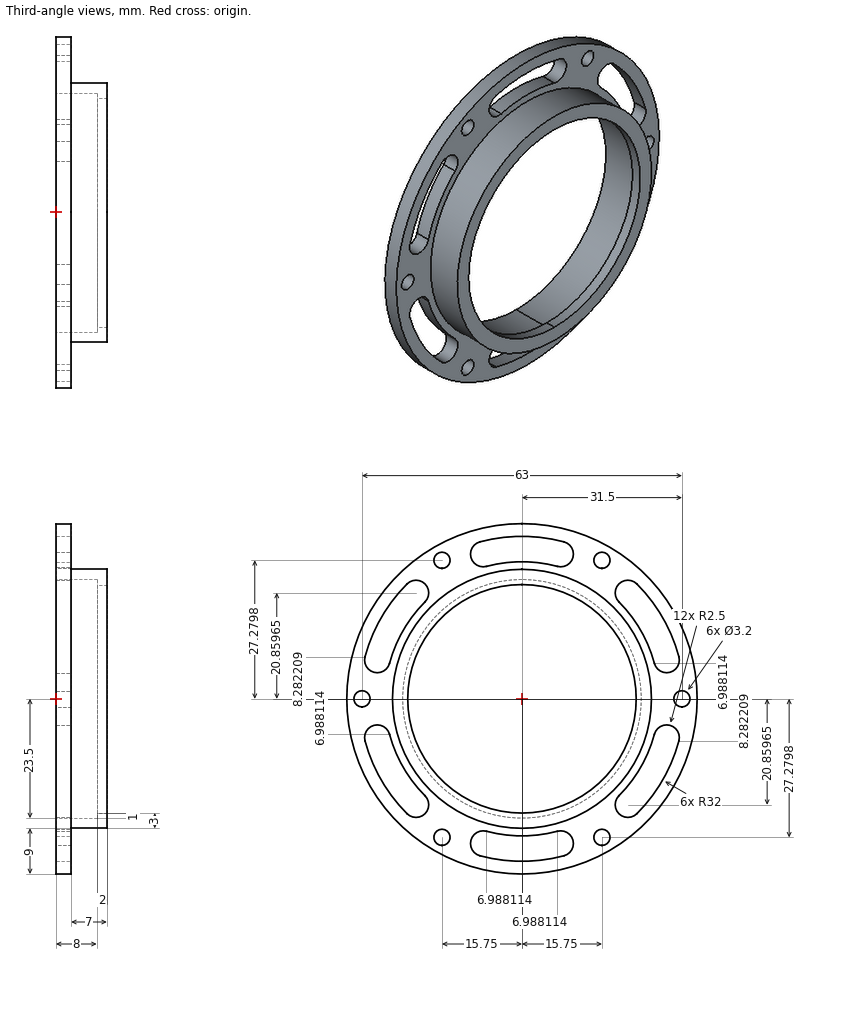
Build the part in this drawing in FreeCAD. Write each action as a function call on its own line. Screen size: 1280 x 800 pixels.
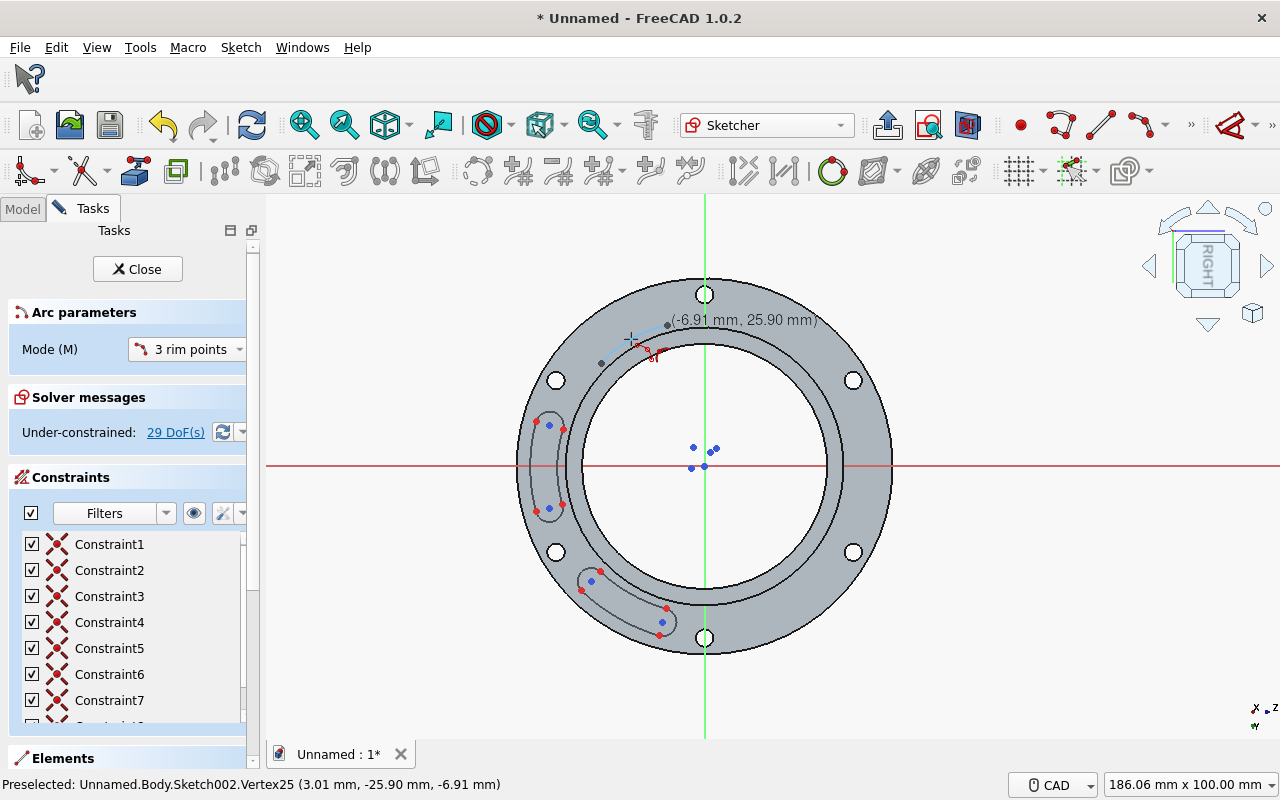
click(660, 298)
click(676, 308)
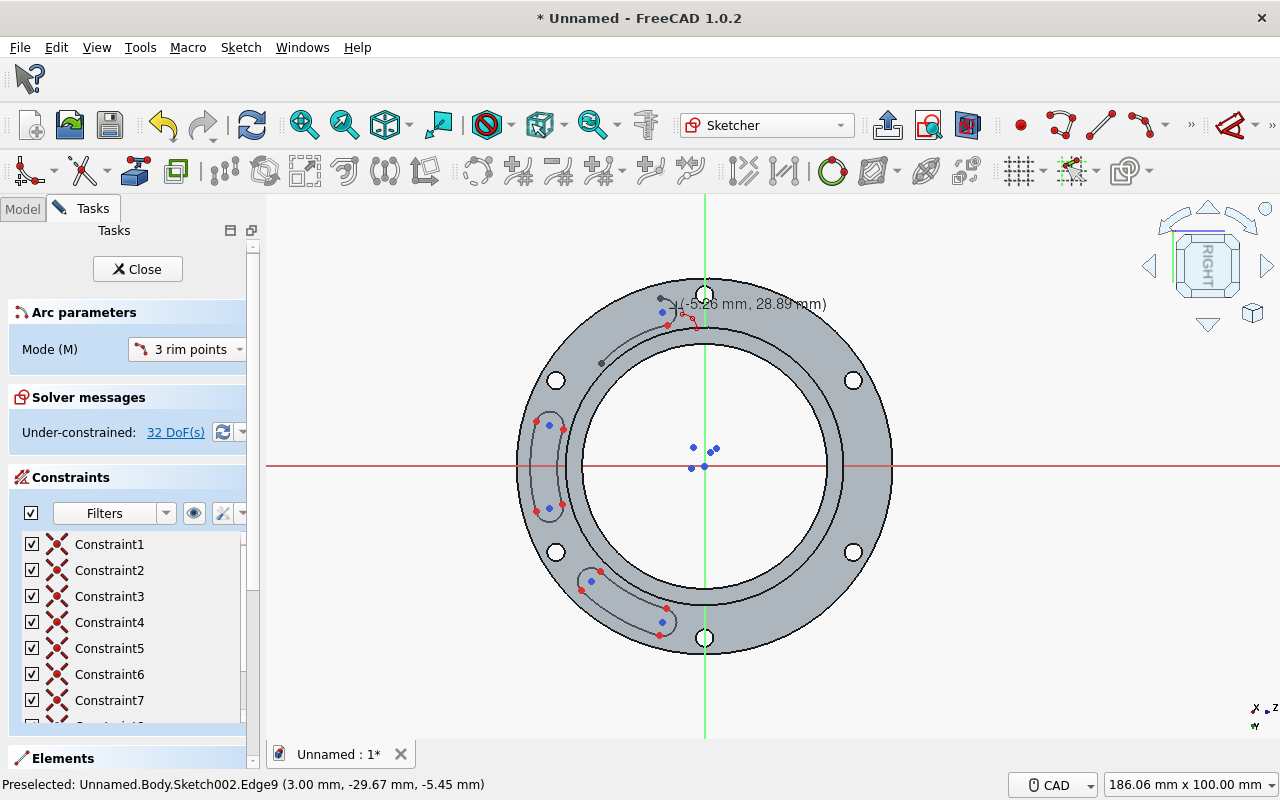
click(660, 299)
click(581, 343)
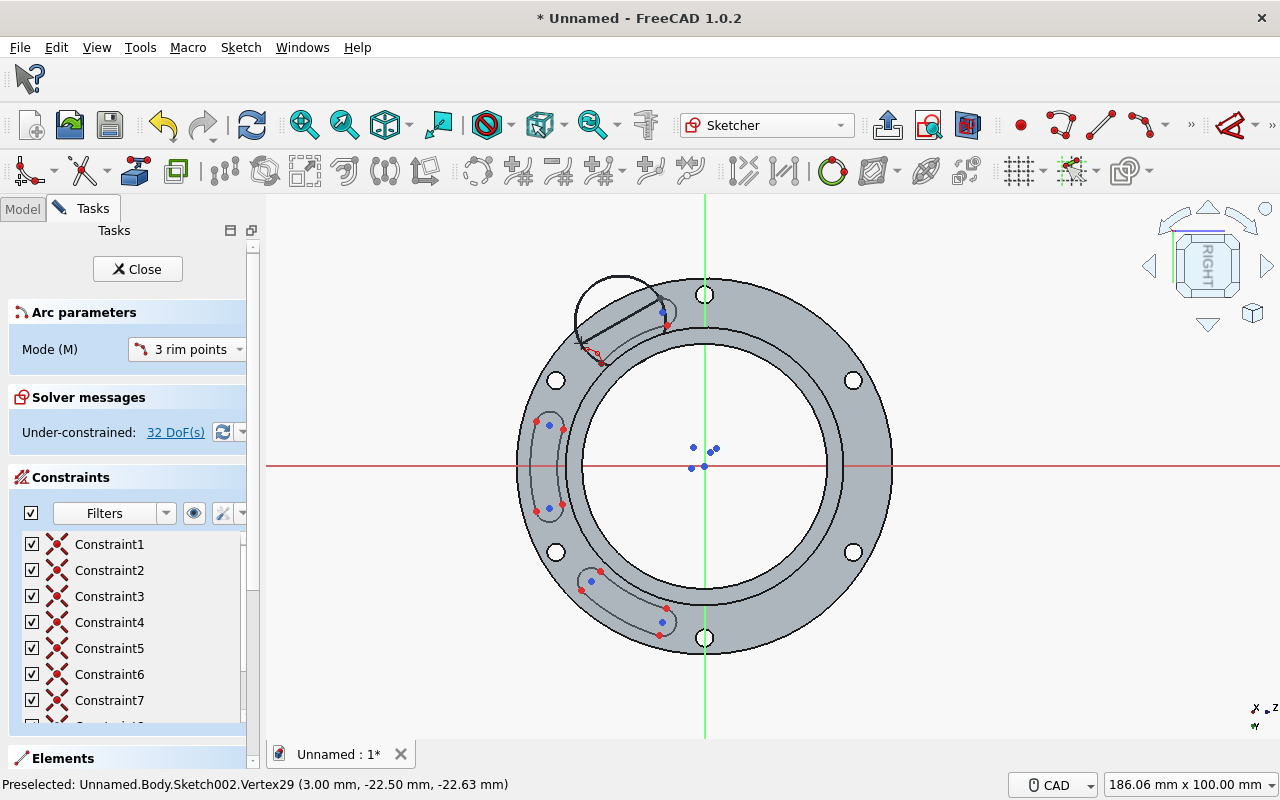
scroll(617, 315, up, 5)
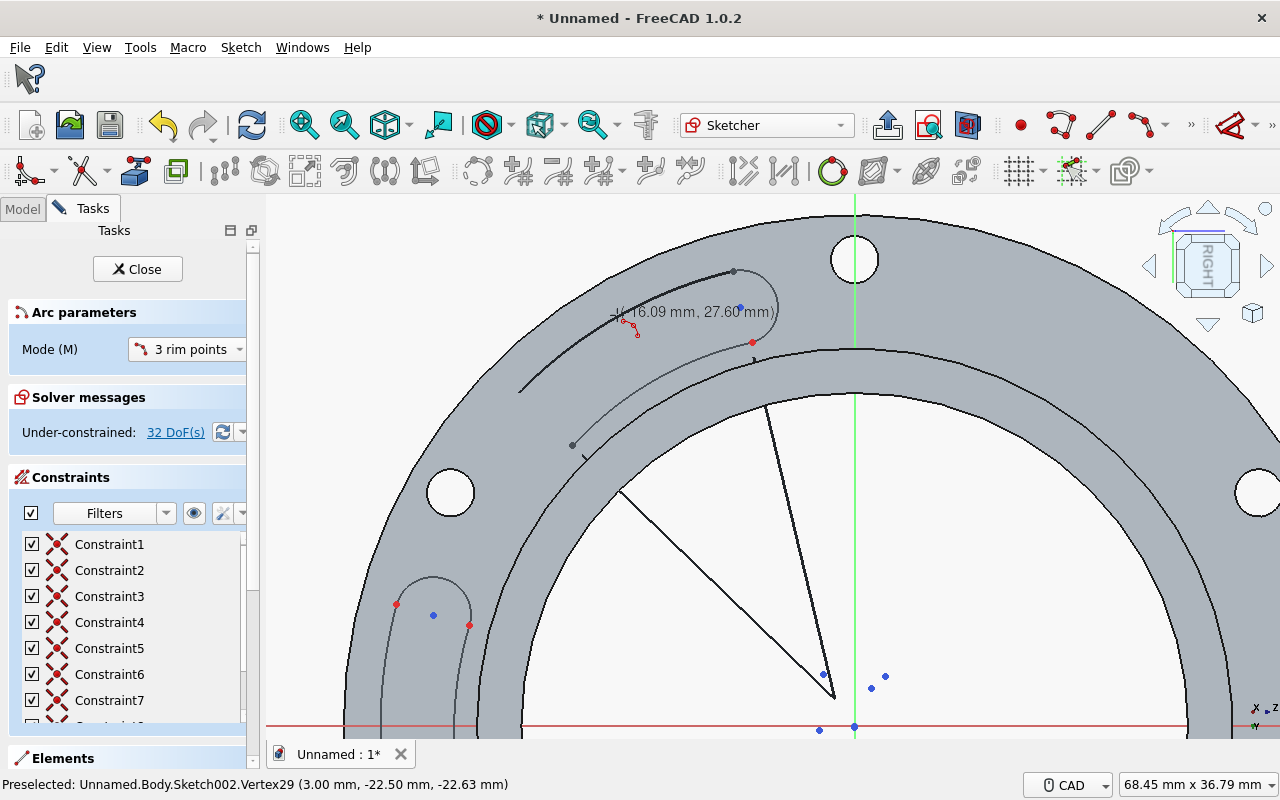
click(618, 316)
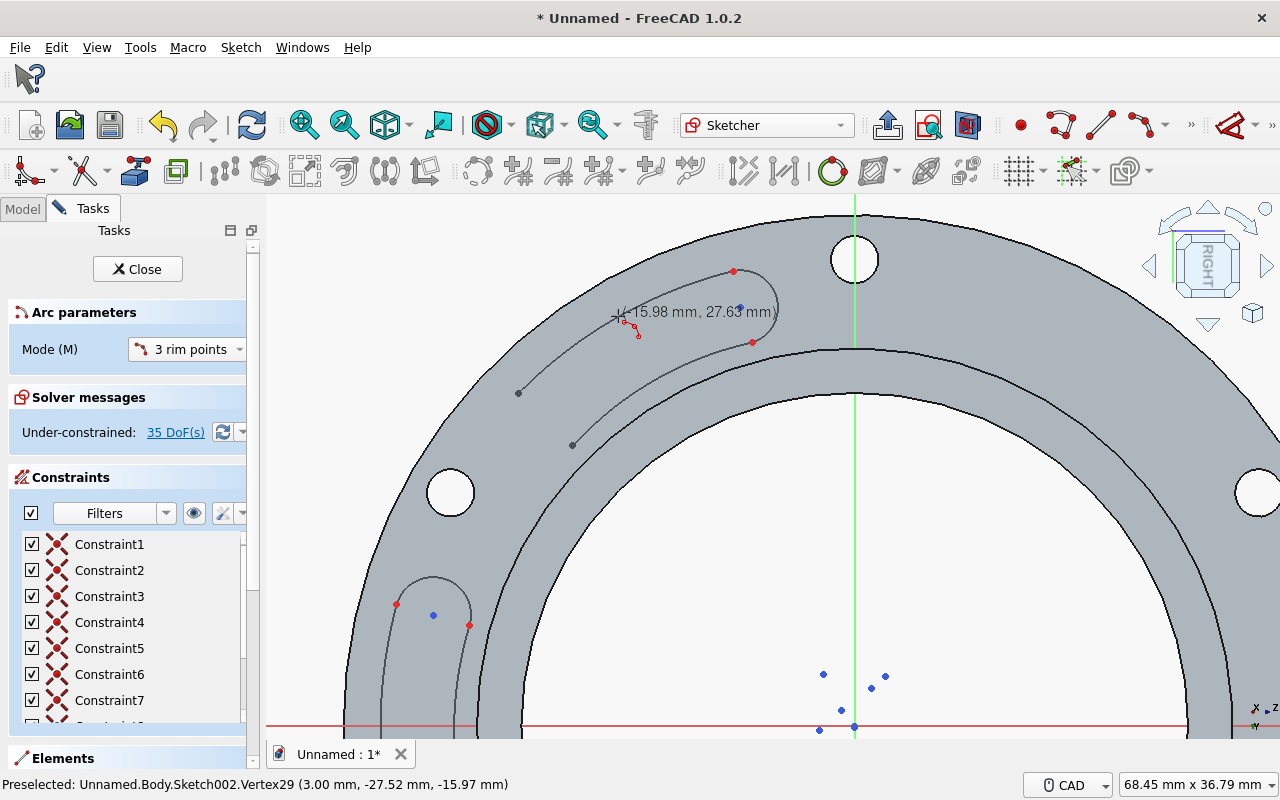
click(519, 393)
click(573, 446)
click(519, 443)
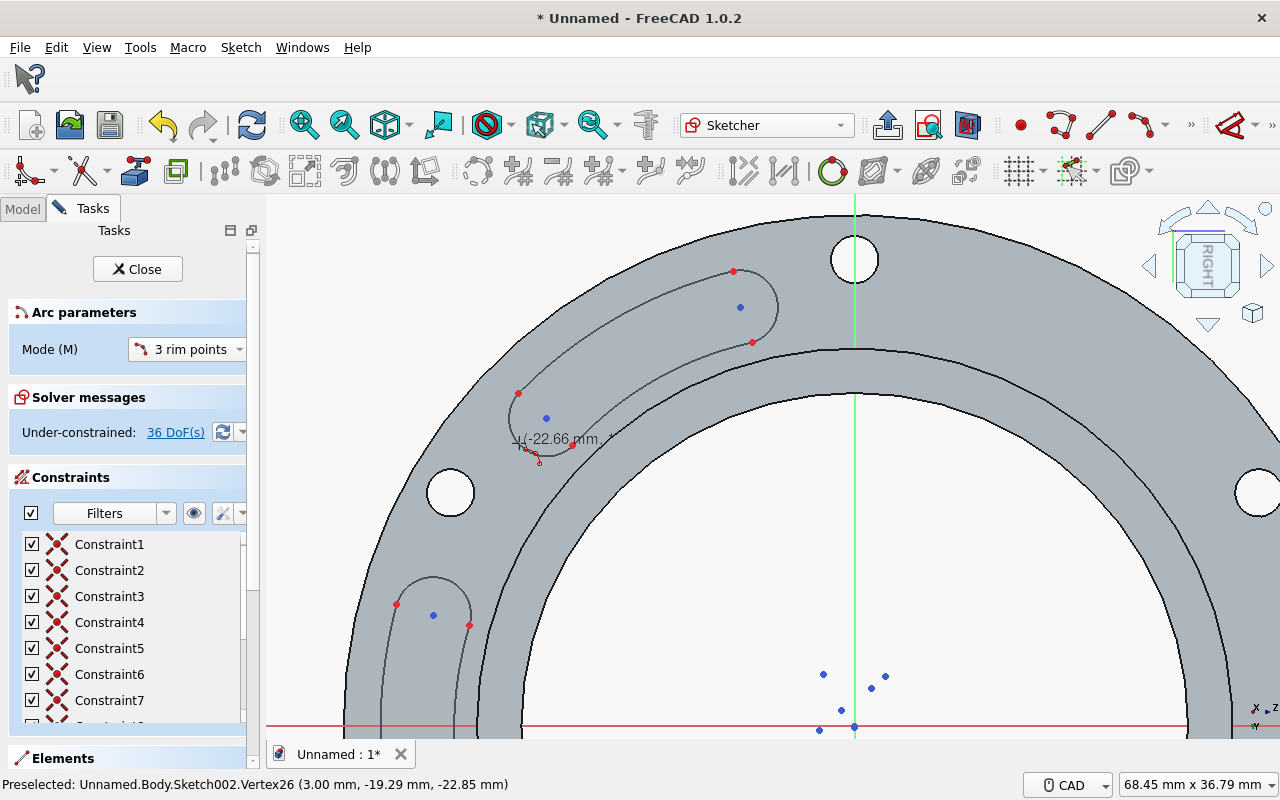
scroll(617, 315, down, 5)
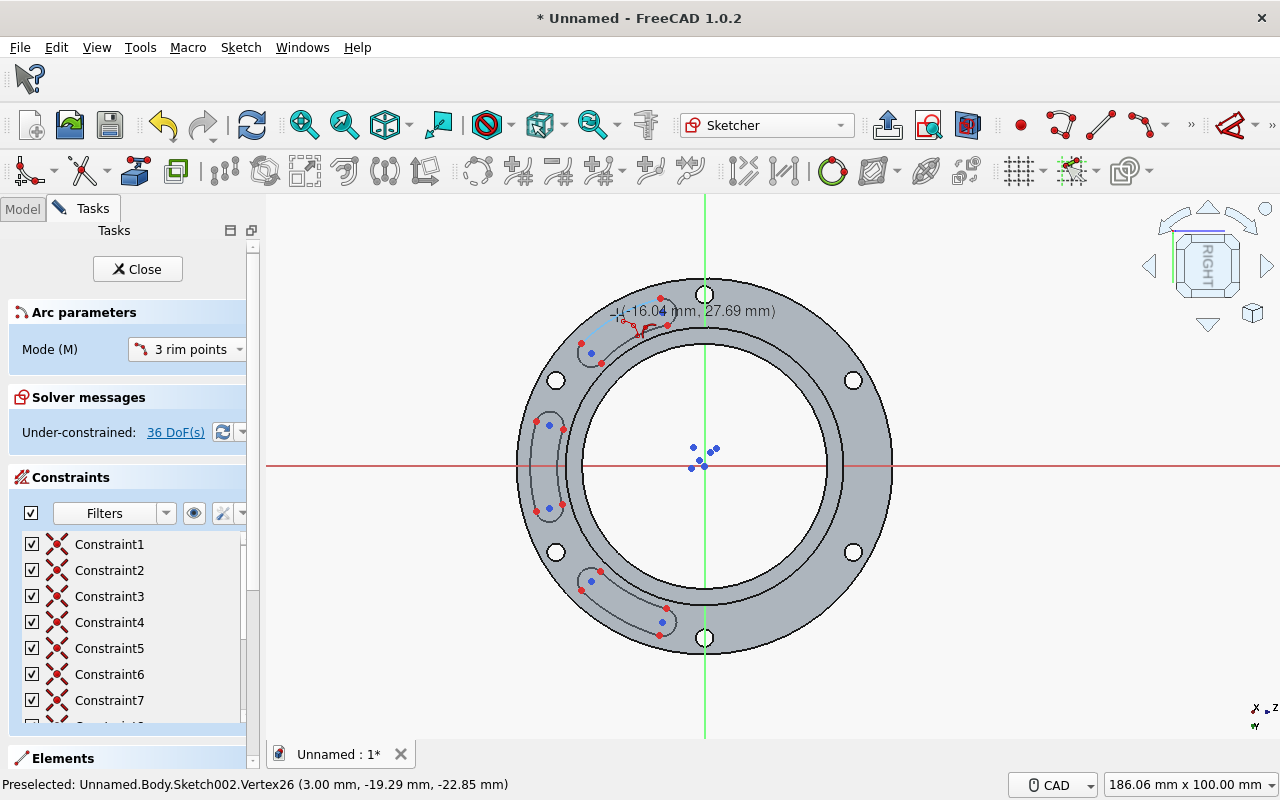
click(809, 362)
click(828, 343)
click(828, 362)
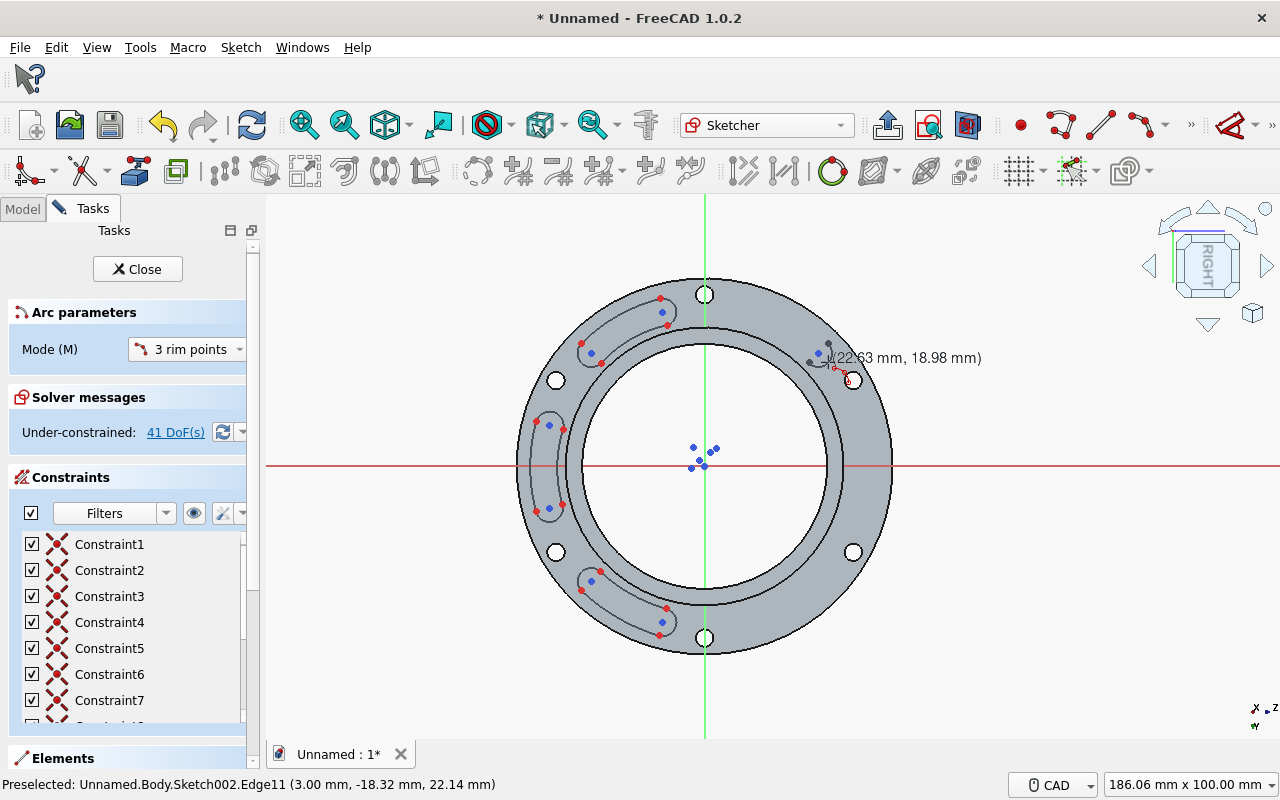
click(828, 344)
click(750, 298)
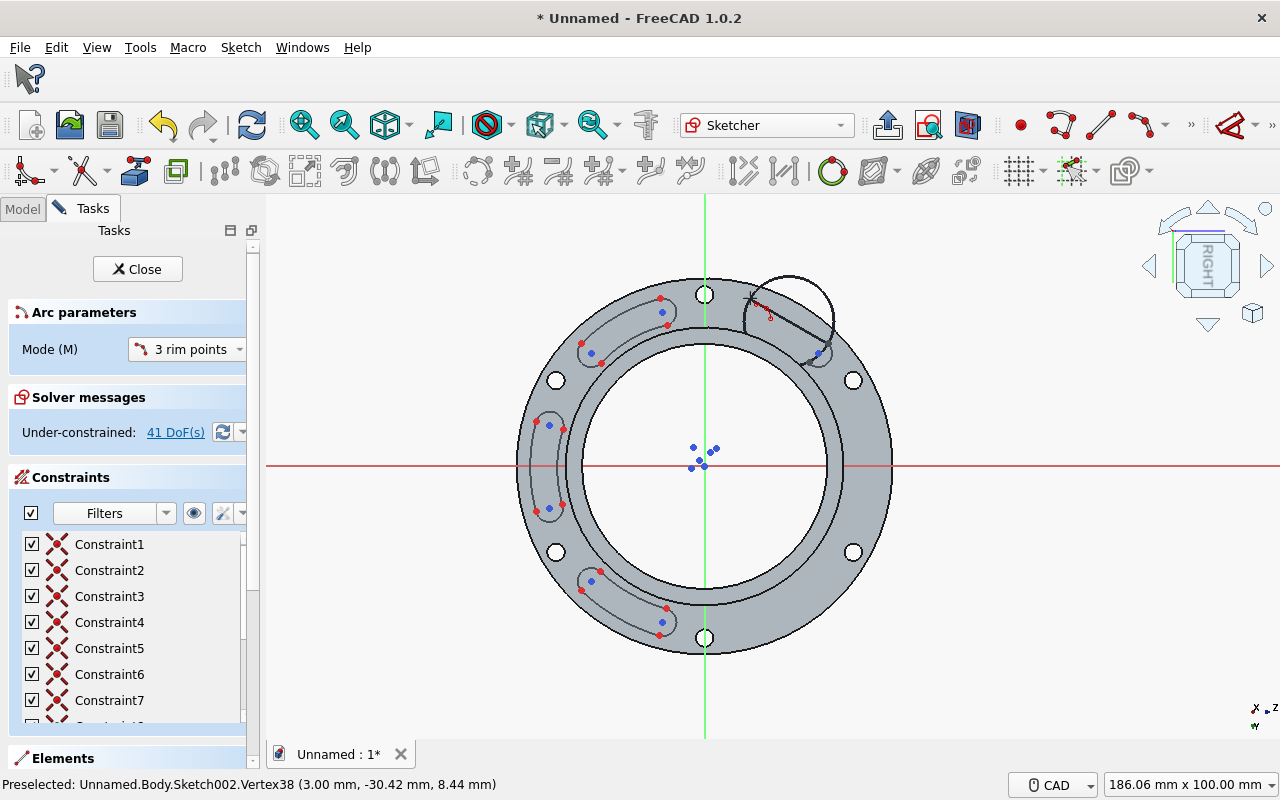
scroll(792, 315, up, 5)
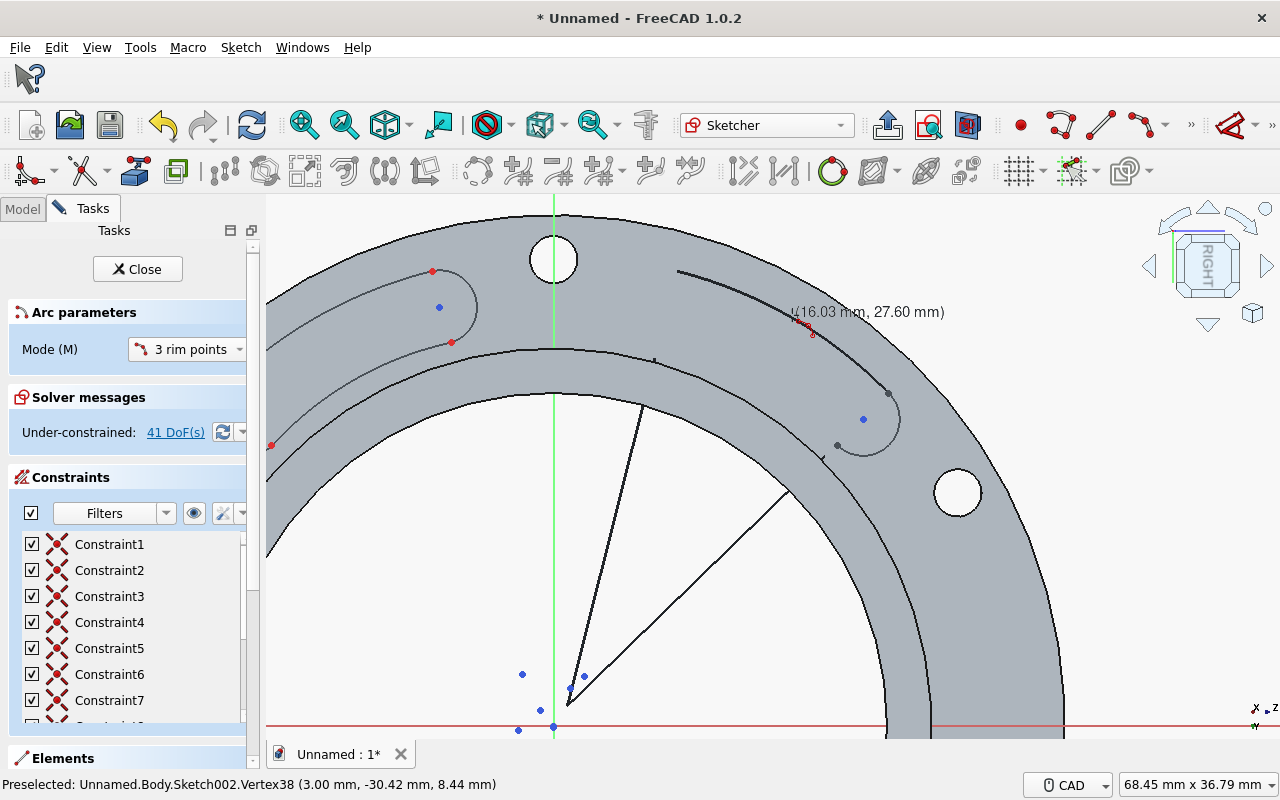
click(791, 316)